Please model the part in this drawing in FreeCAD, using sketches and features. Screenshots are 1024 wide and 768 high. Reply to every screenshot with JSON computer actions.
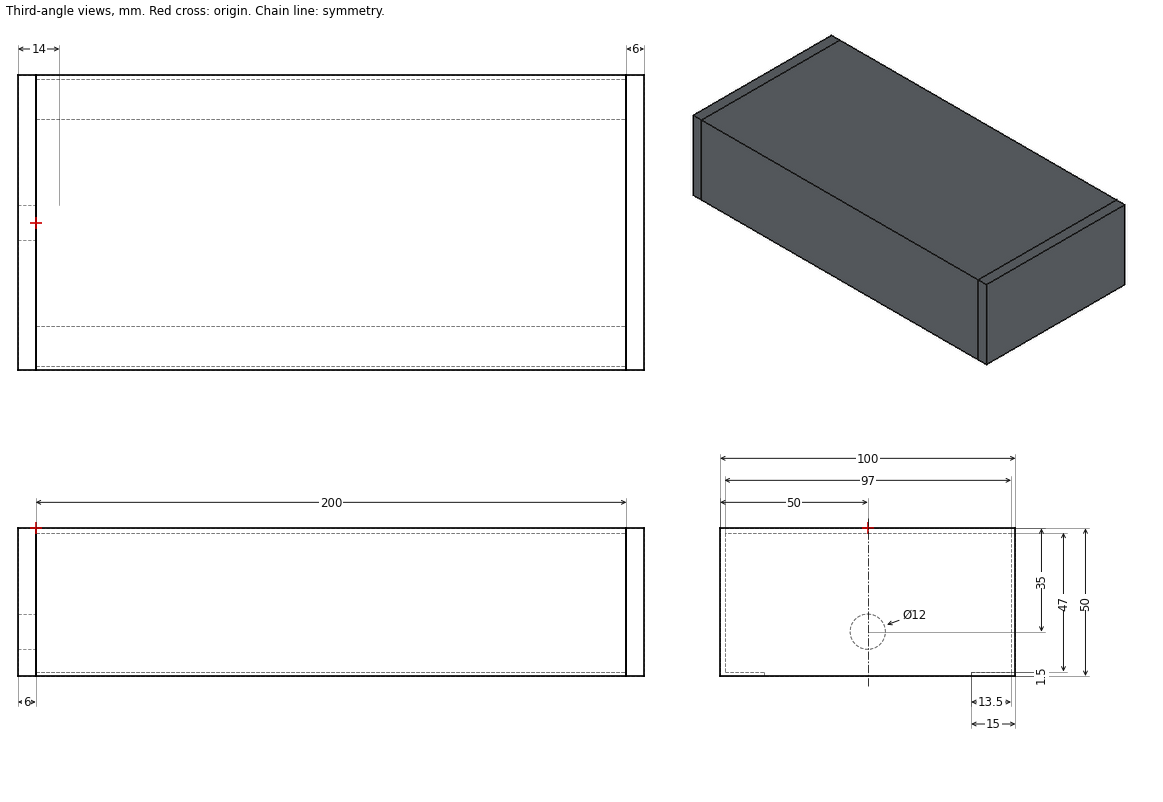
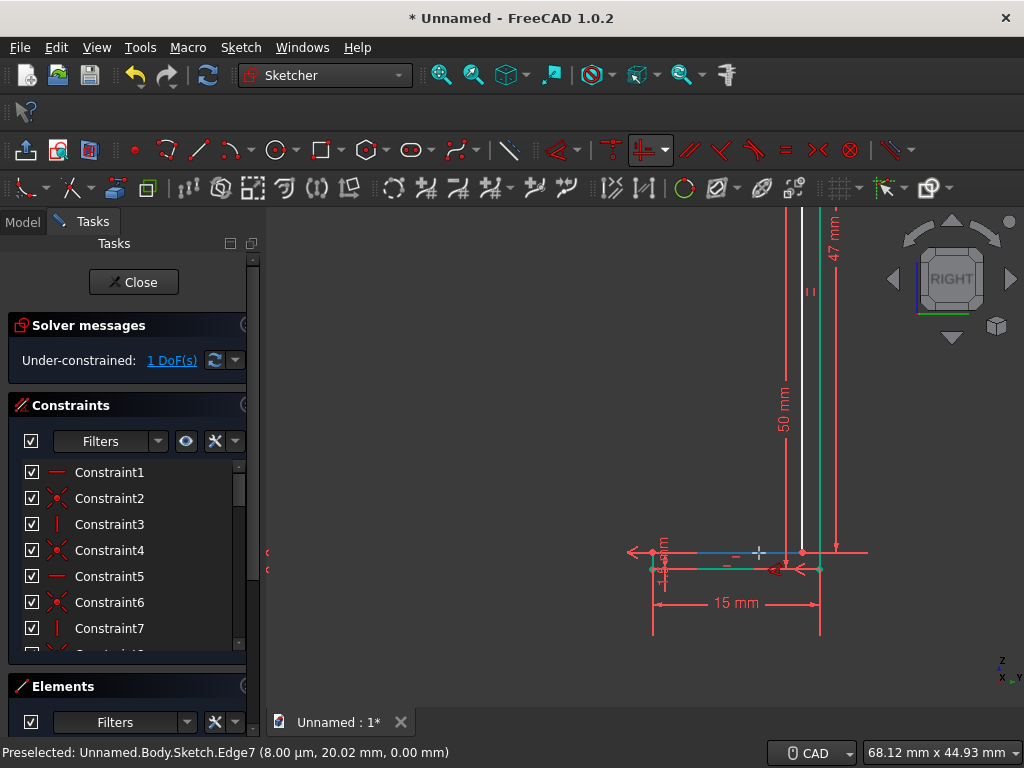
{"action": "left_click", "coordinate": [758, 553]}
{"action": "left_click", "coordinate": [728, 519]}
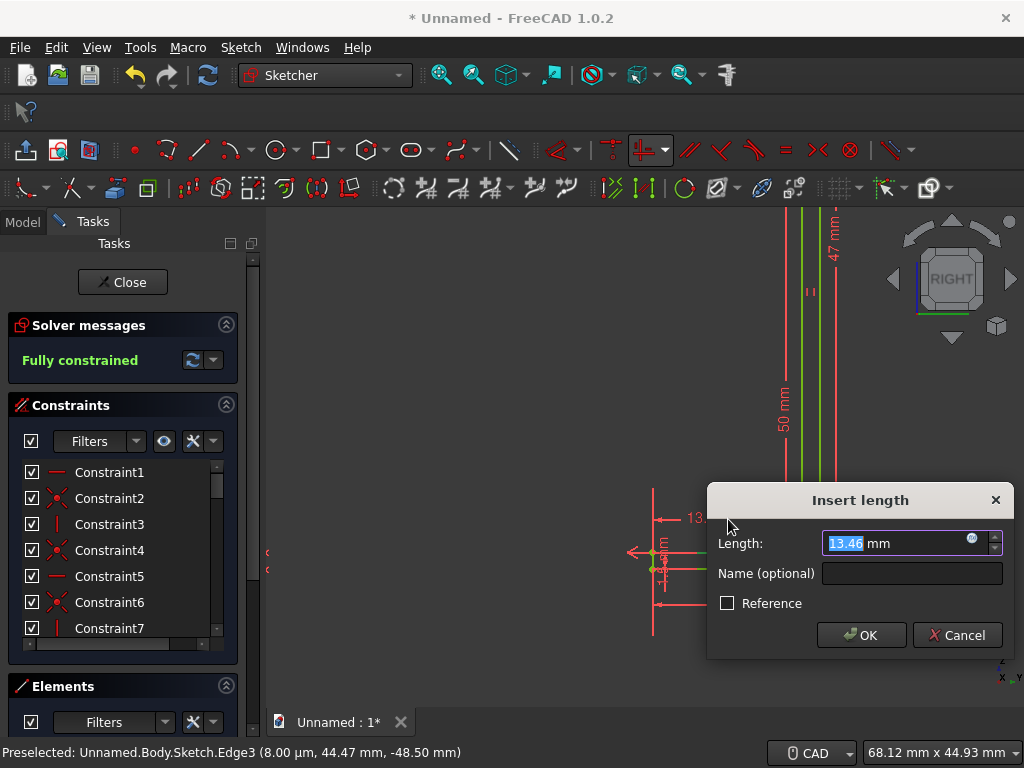
{"action": "type", "text": "13.5"}
{"action": "key", "text": "Return"}
{"action": "key", "text": "Escape"}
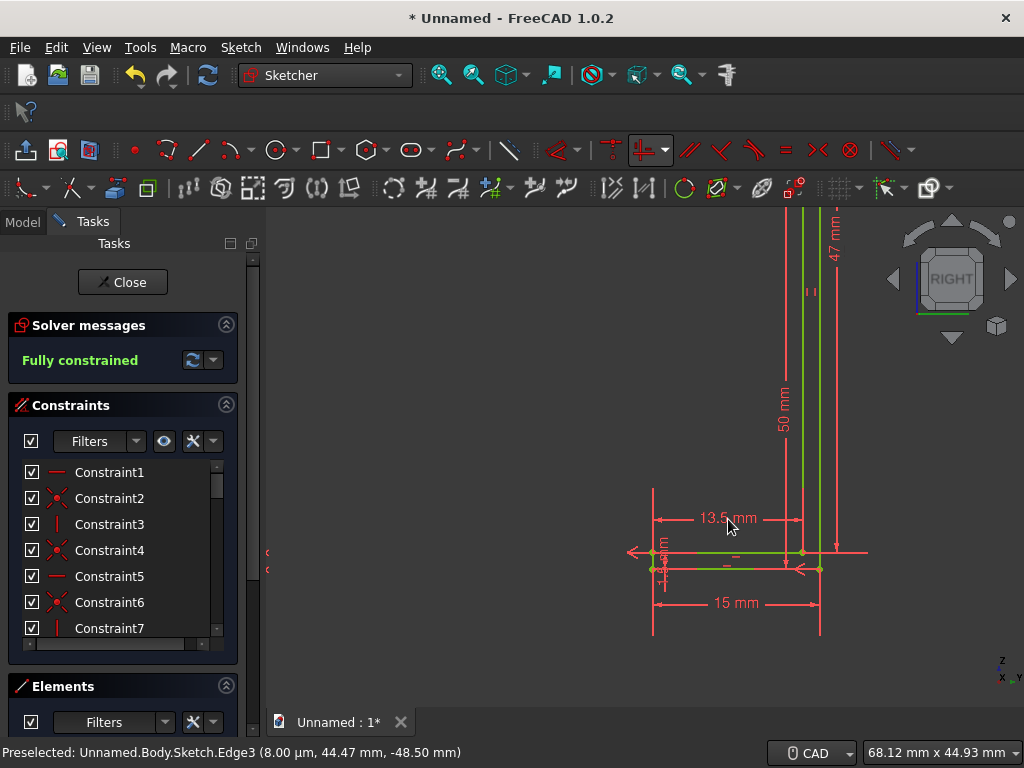
{"action": "left_click", "coordinate": [123, 282]}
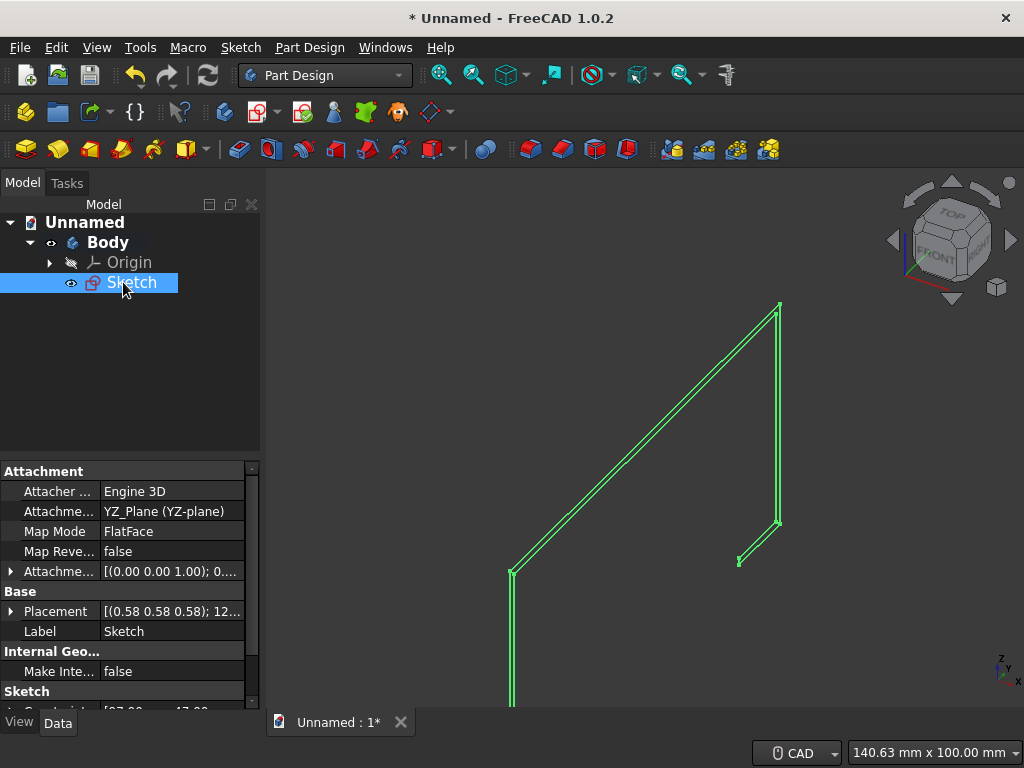
{"action": "left_click", "coordinate": [26, 150]}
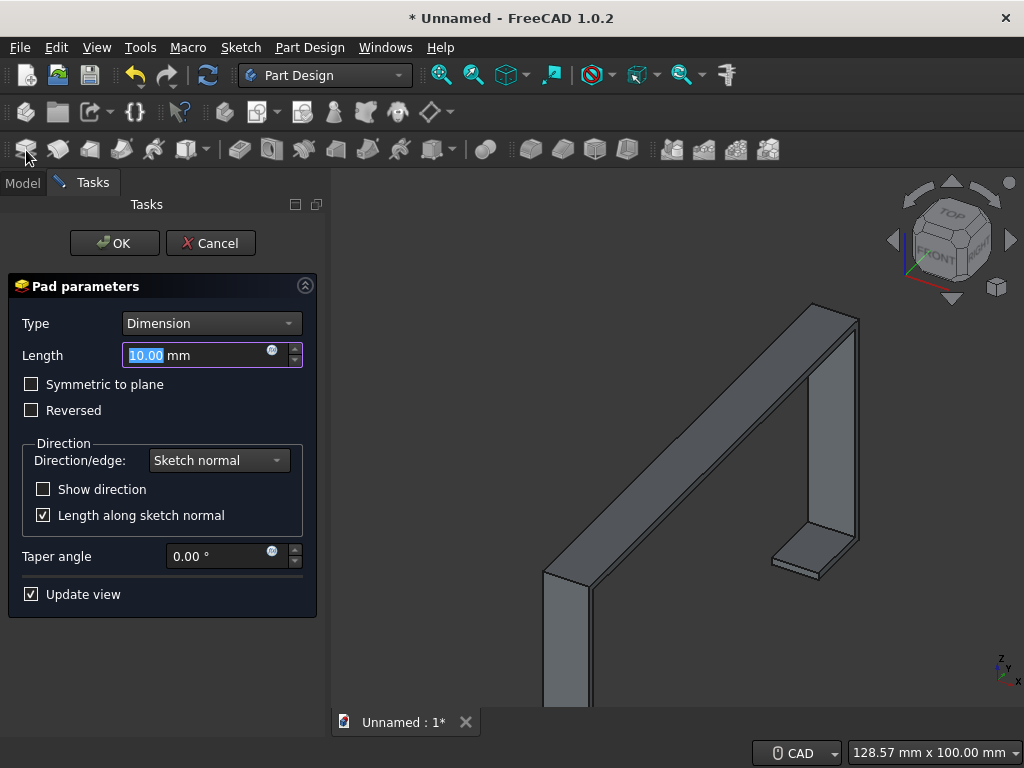
{"action": "type", "text": "200"}
{"action": "key", "text": "Tab"}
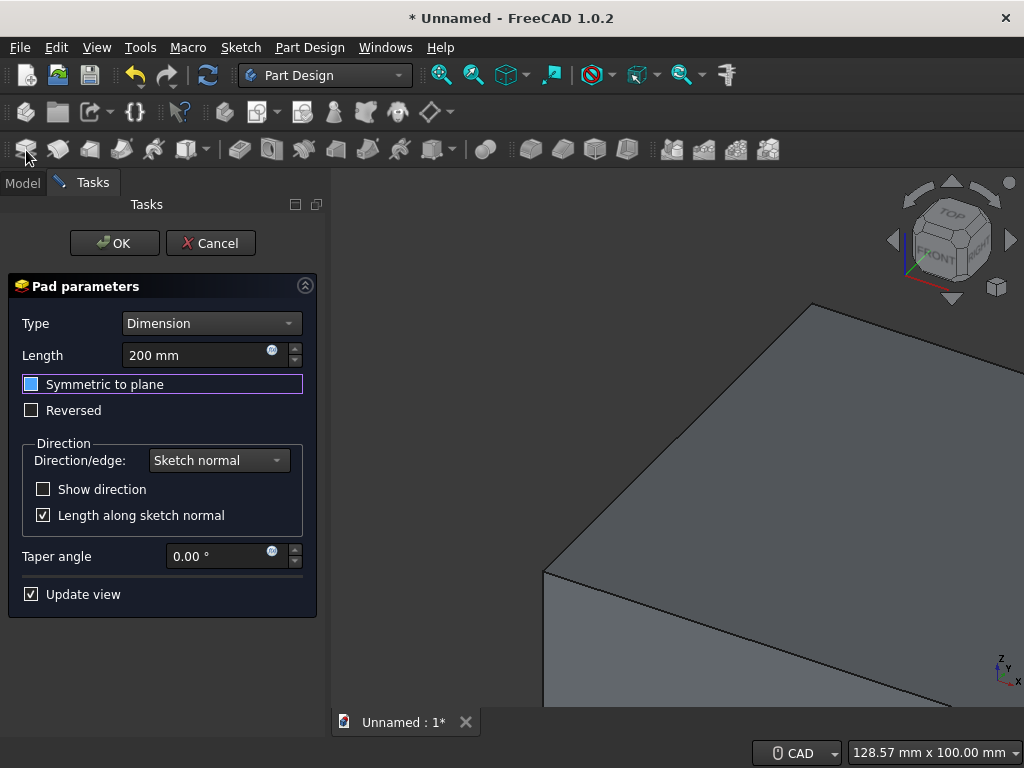
{"action": "left_click", "coordinate": [115, 243]}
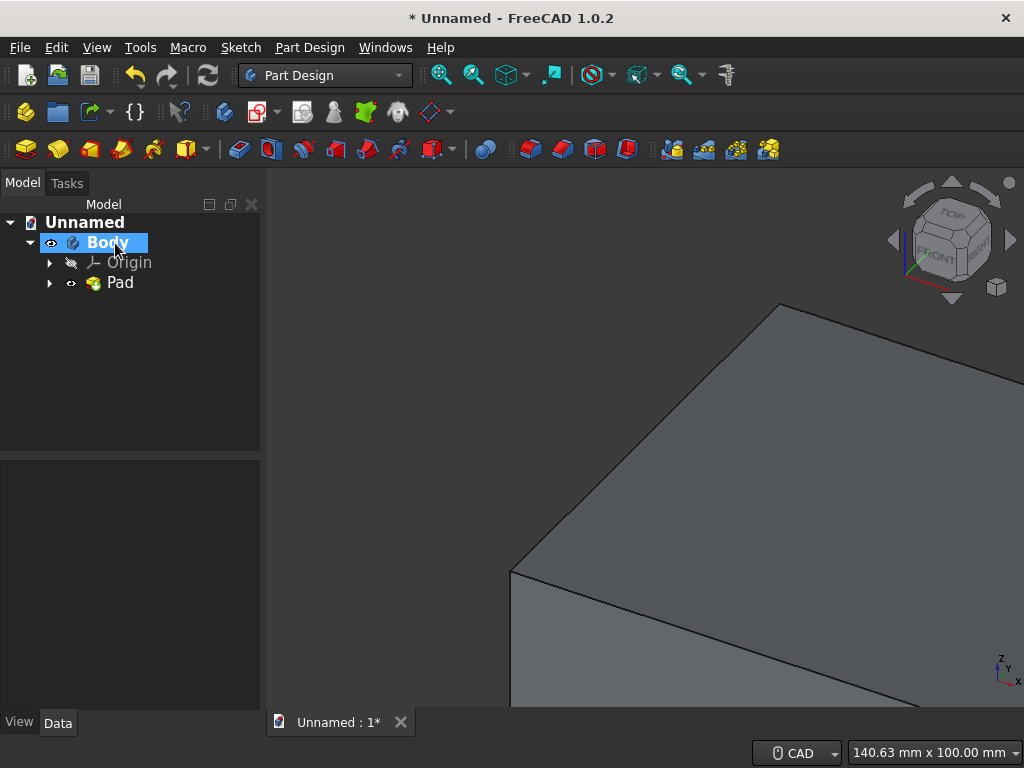
{"action": "key", "text": "v f"}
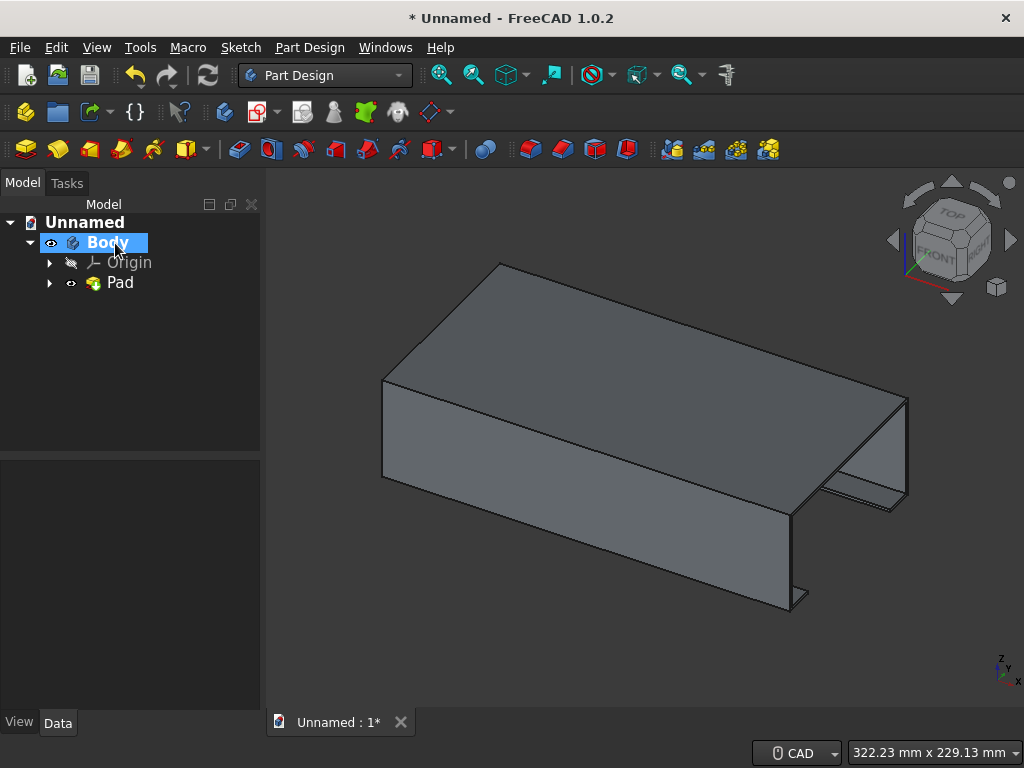
{"action": "left_click", "coordinate": [226, 112]}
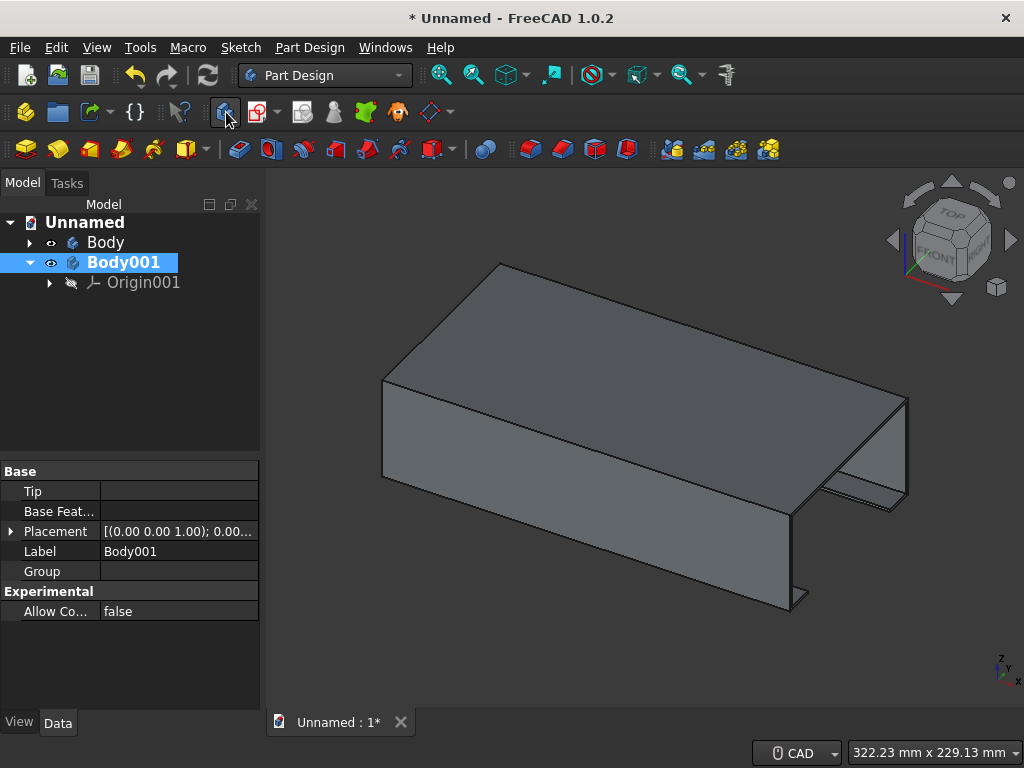
{"action": "left_click", "coordinate": [50, 283]}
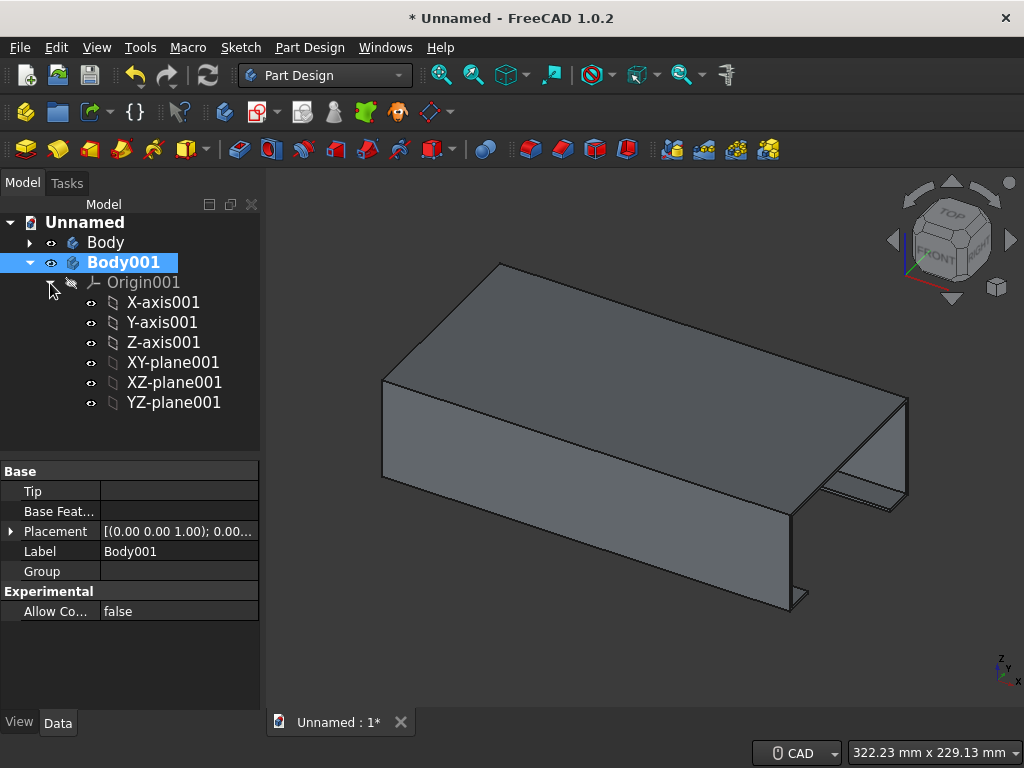
{"action": "left_click", "coordinate": [136, 403]}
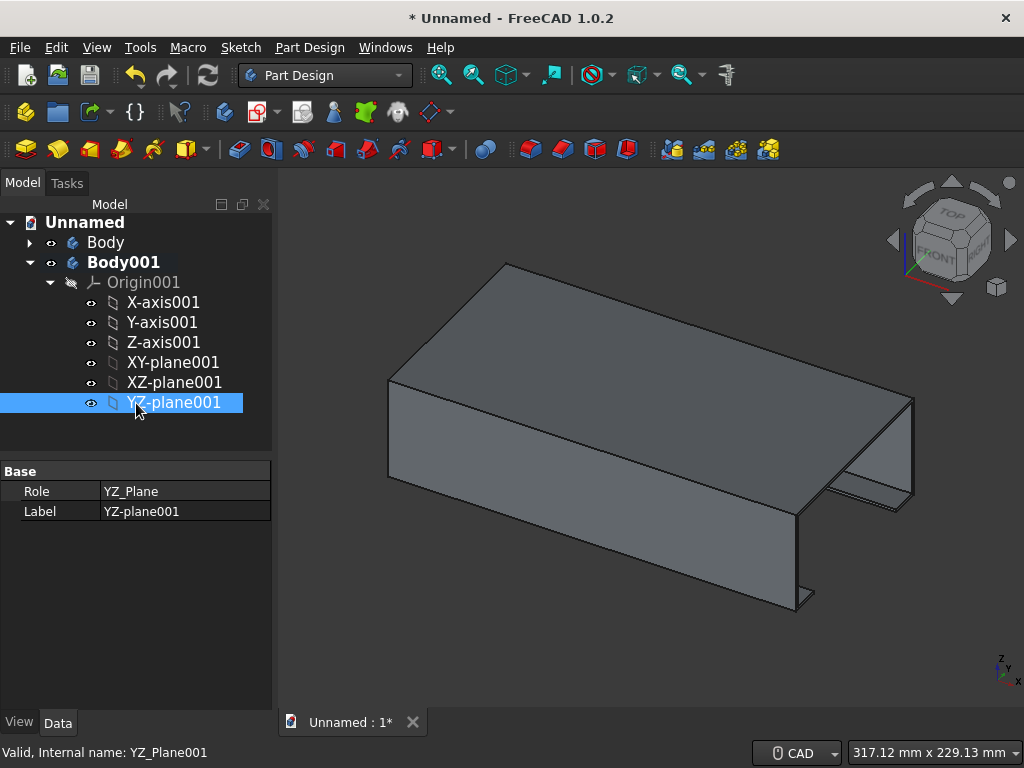
{"action": "left_click", "coordinate": [430, 112]}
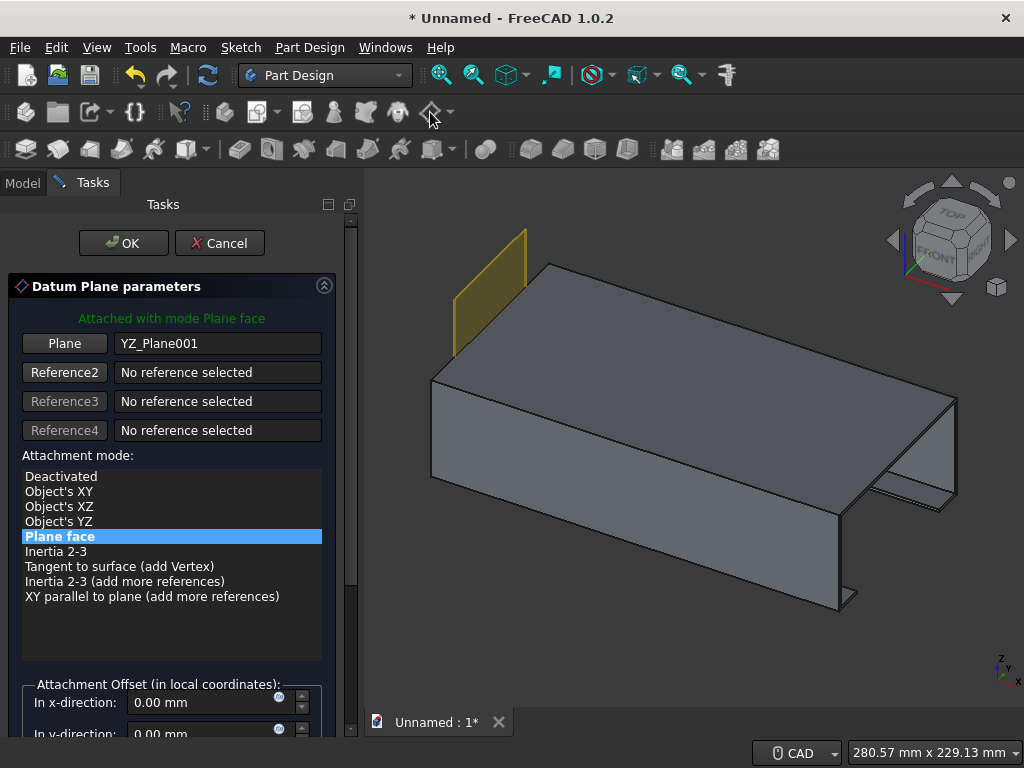
{"action": "scroll", "coordinate": [351, 475], "scroll_direction": "down", "scroll_amount": 2}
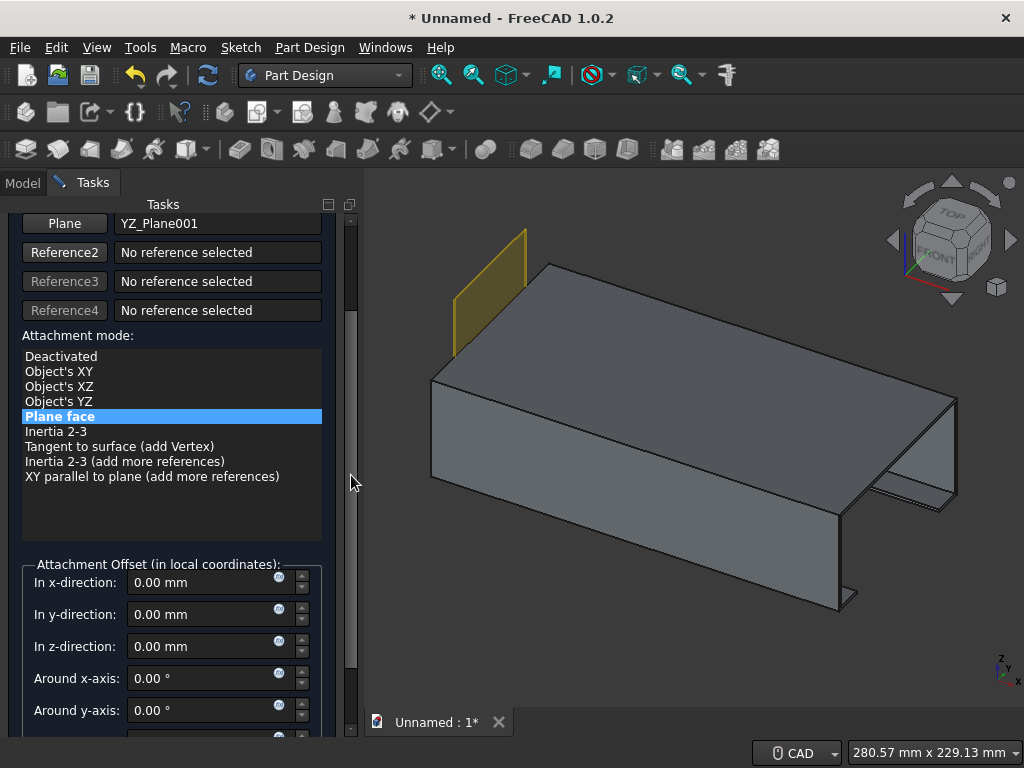
{"action": "triple_click", "coordinate": [210, 646]}